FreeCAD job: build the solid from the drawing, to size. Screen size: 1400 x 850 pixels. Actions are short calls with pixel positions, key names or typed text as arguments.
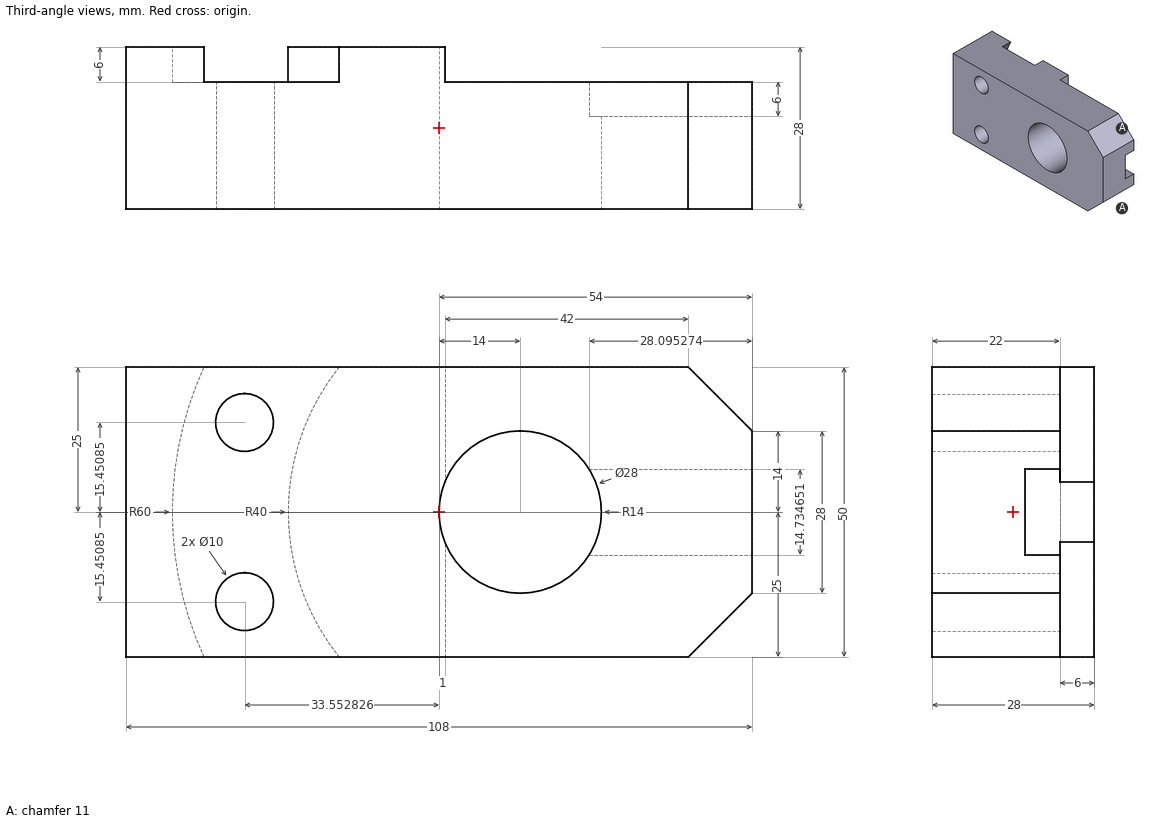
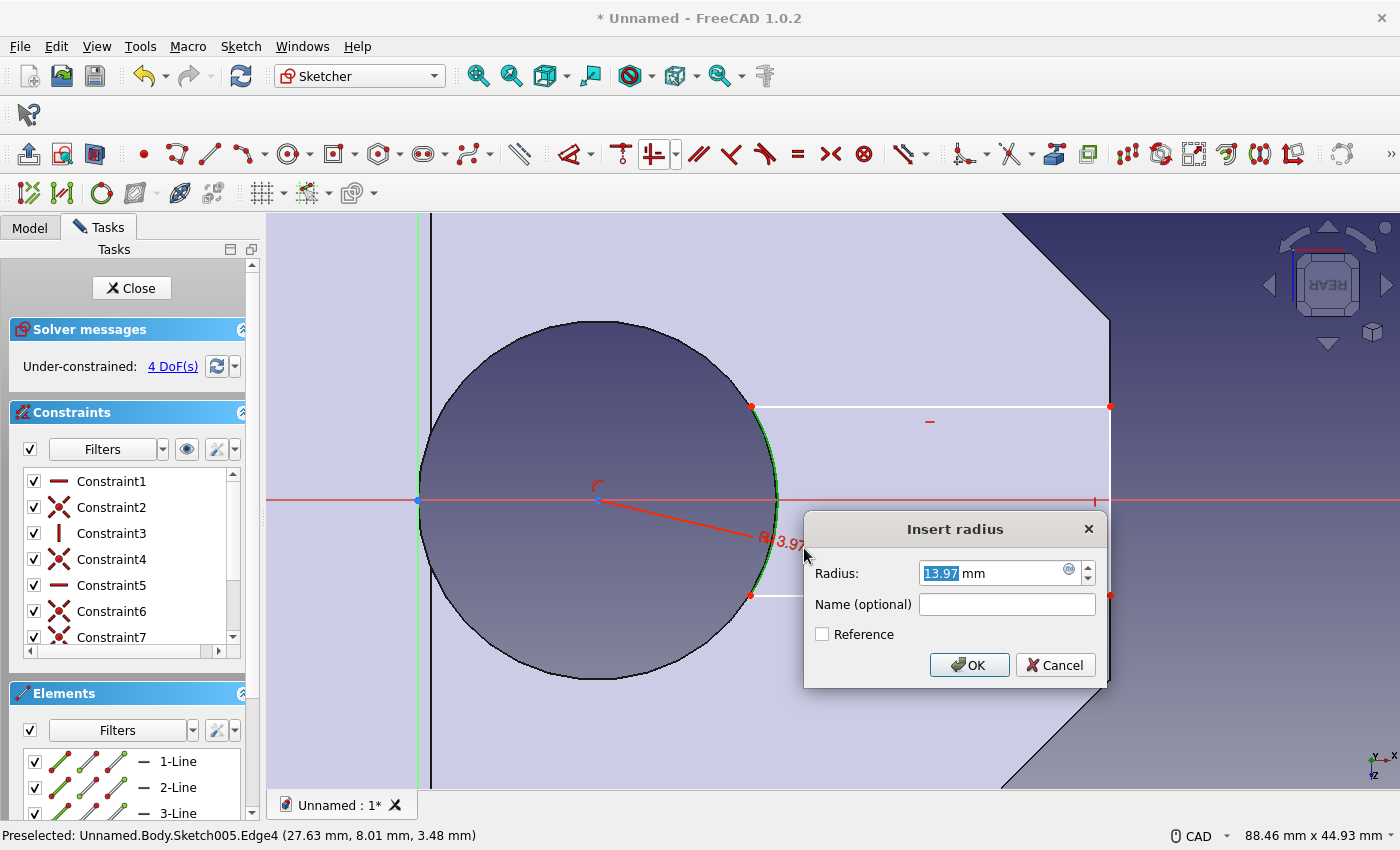
text(14)
key(Return)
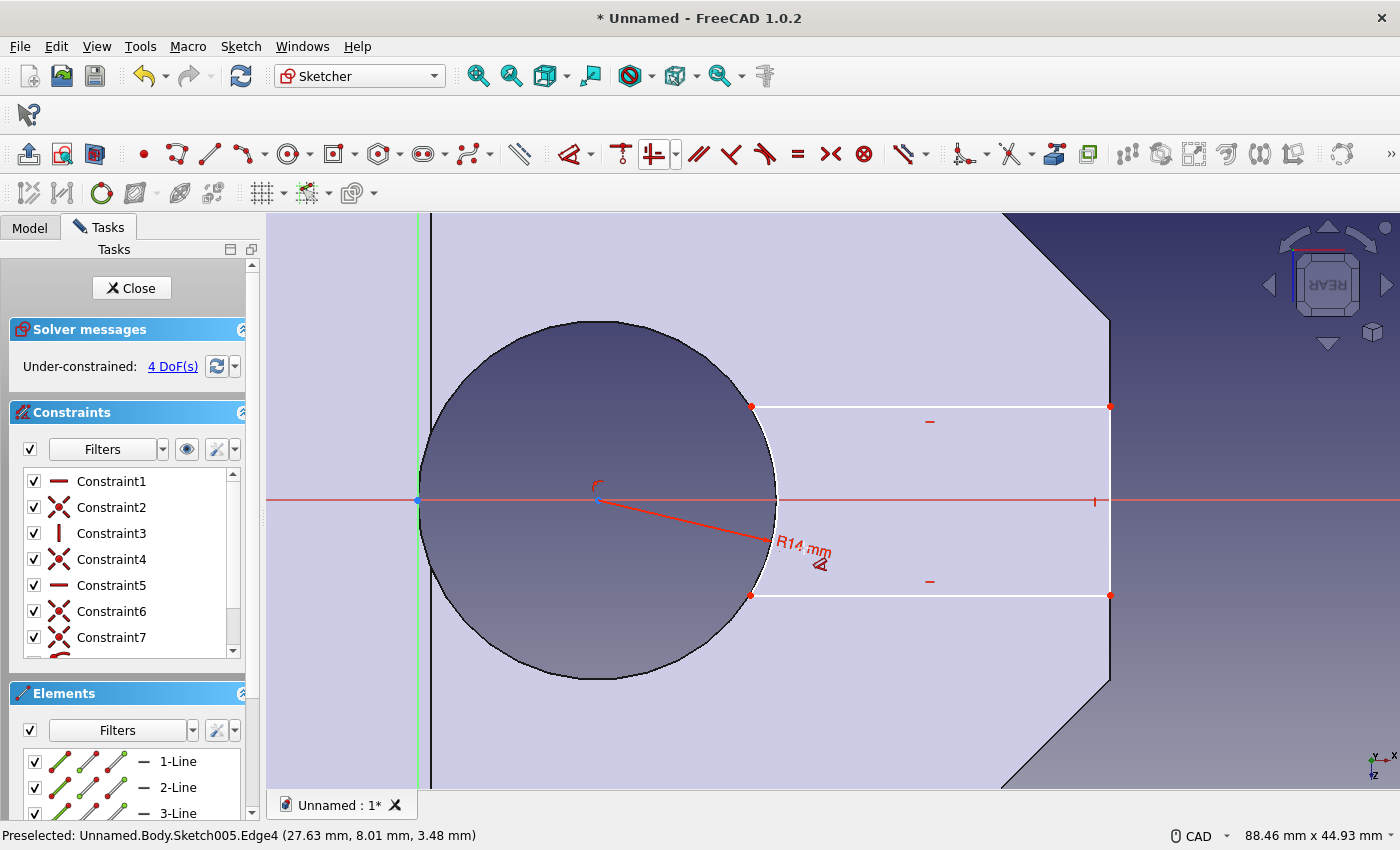
click(1110, 596)
click(764, 630)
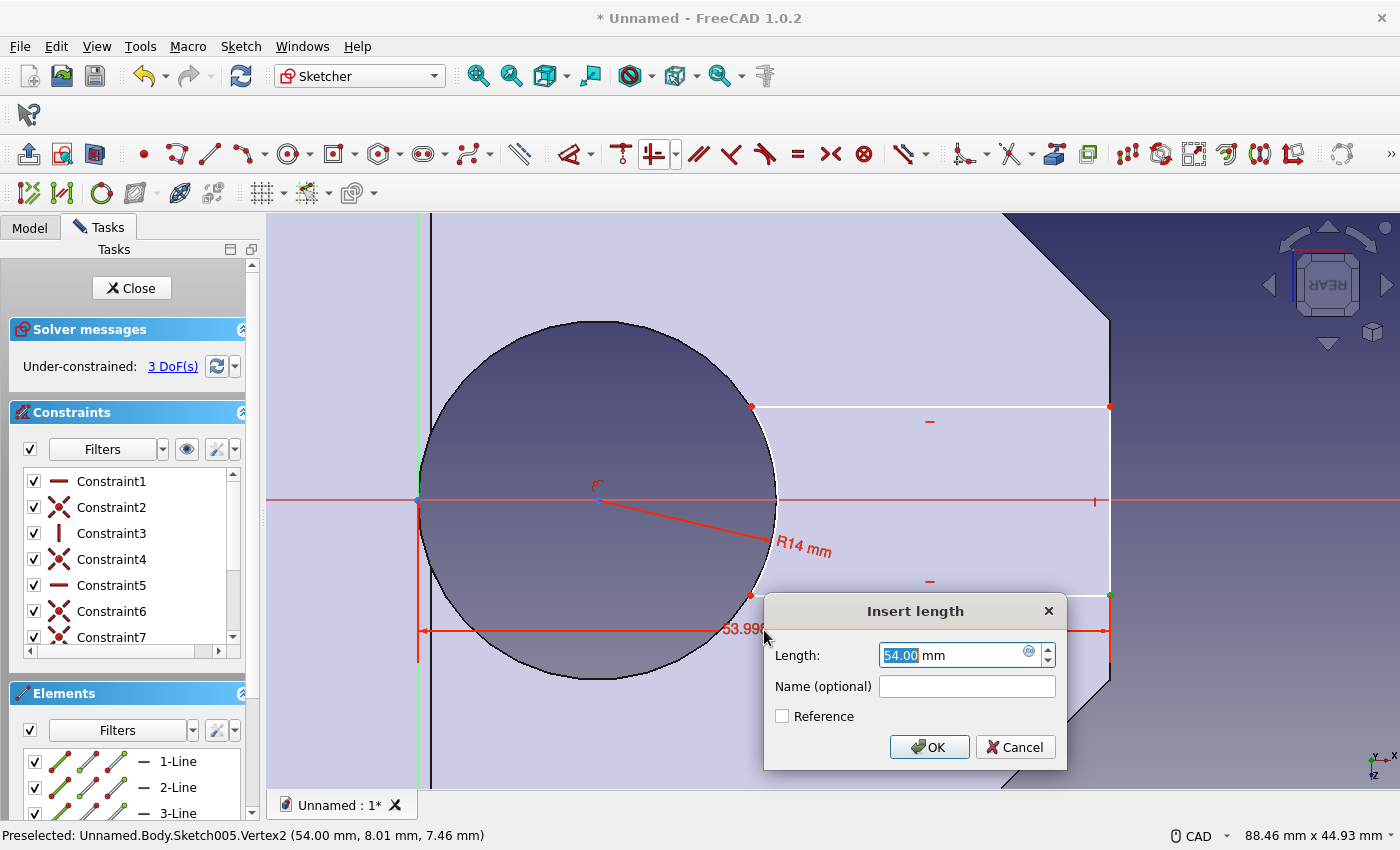
text(54)
key(Return)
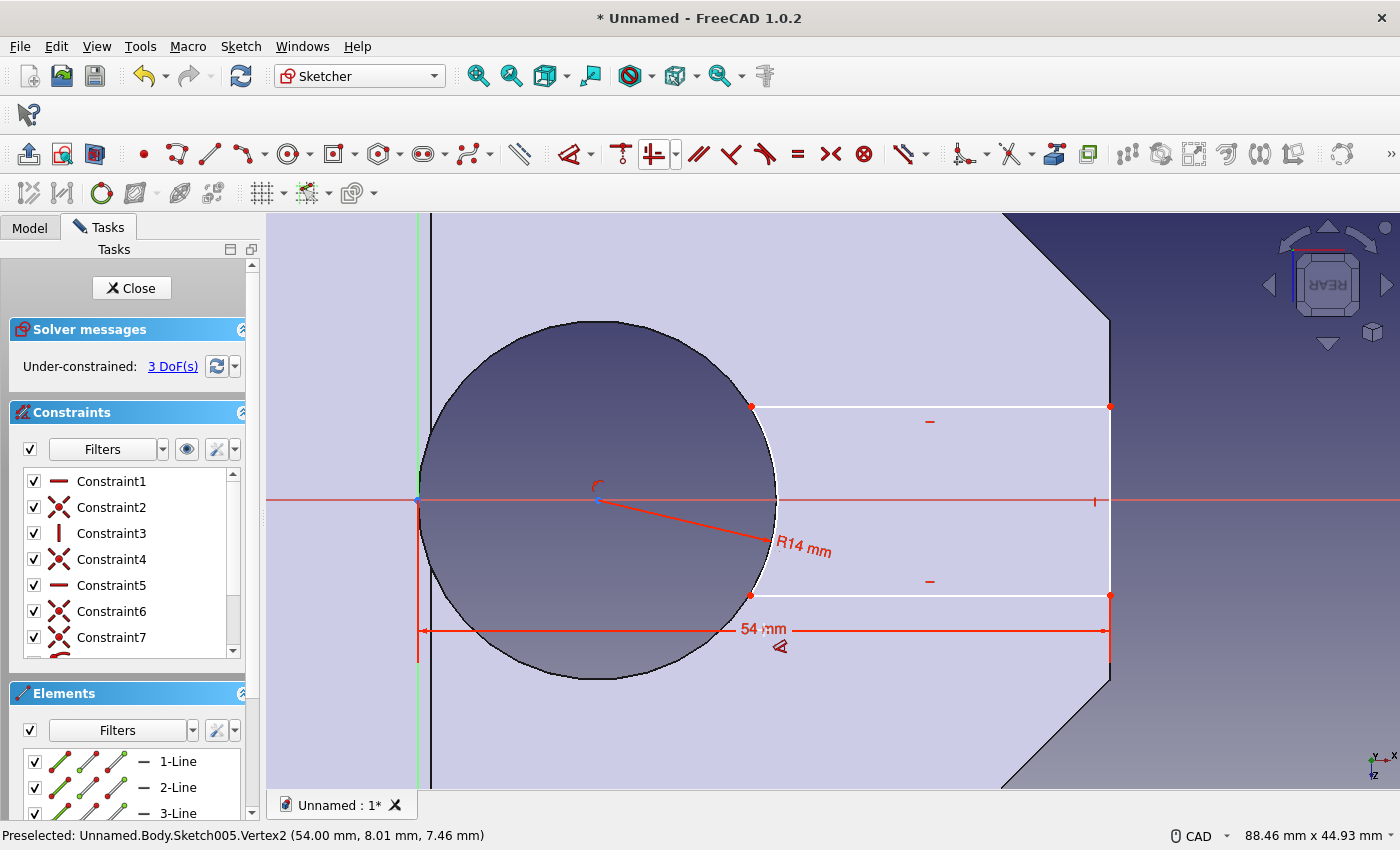
click(598, 500)
click(508, 534)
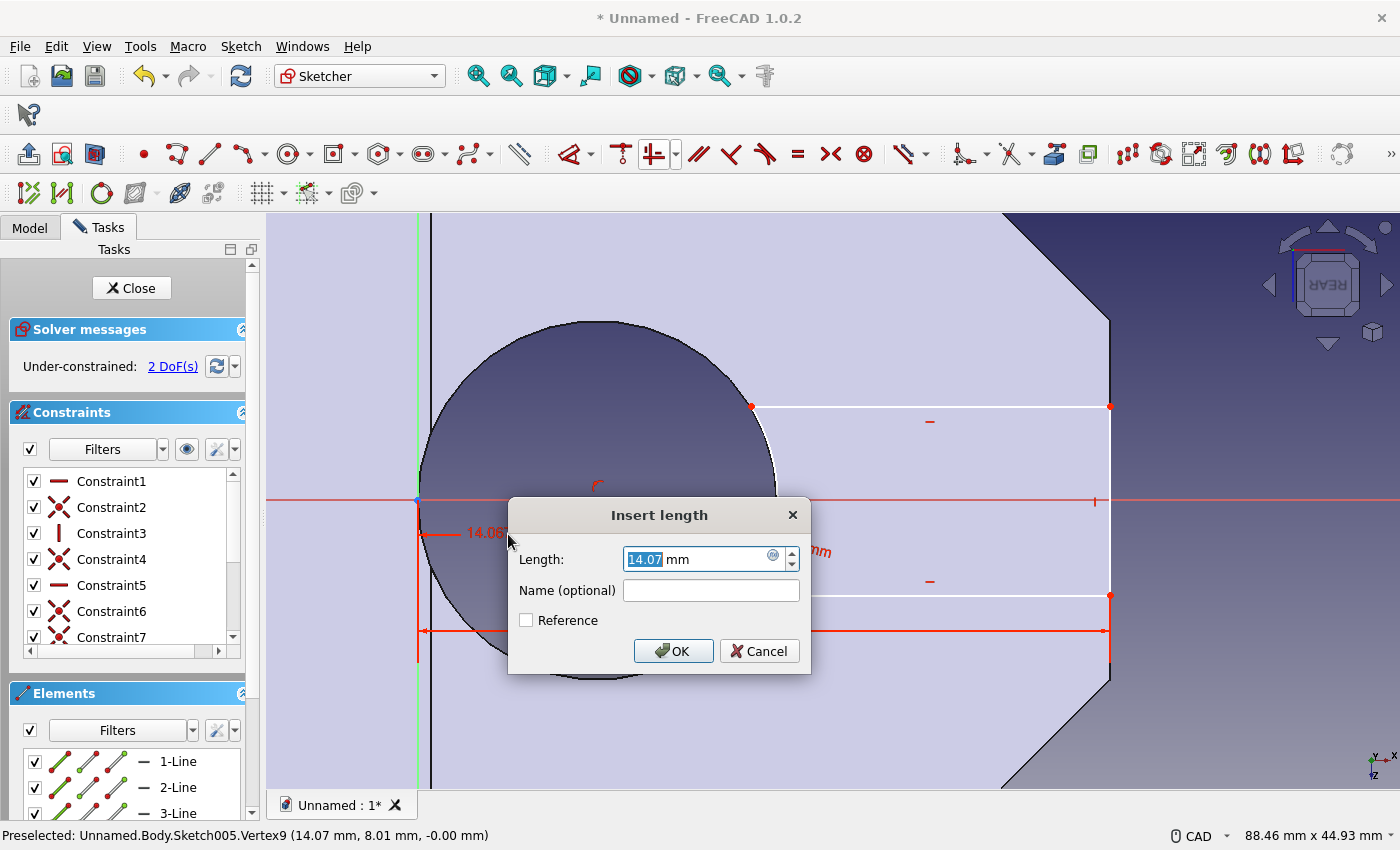
text(14)
key(Return)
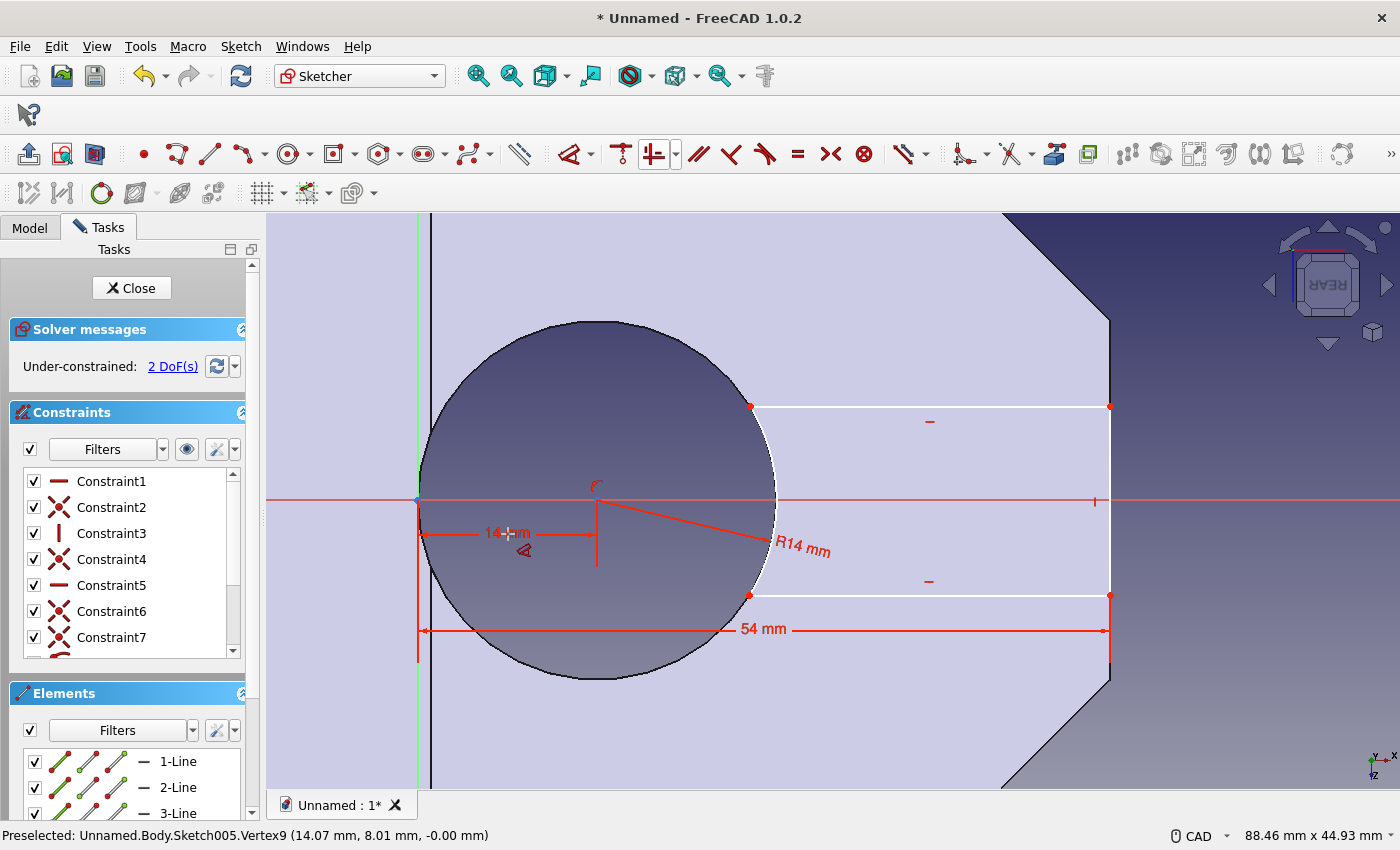
click(857, 596)
click(930, 630)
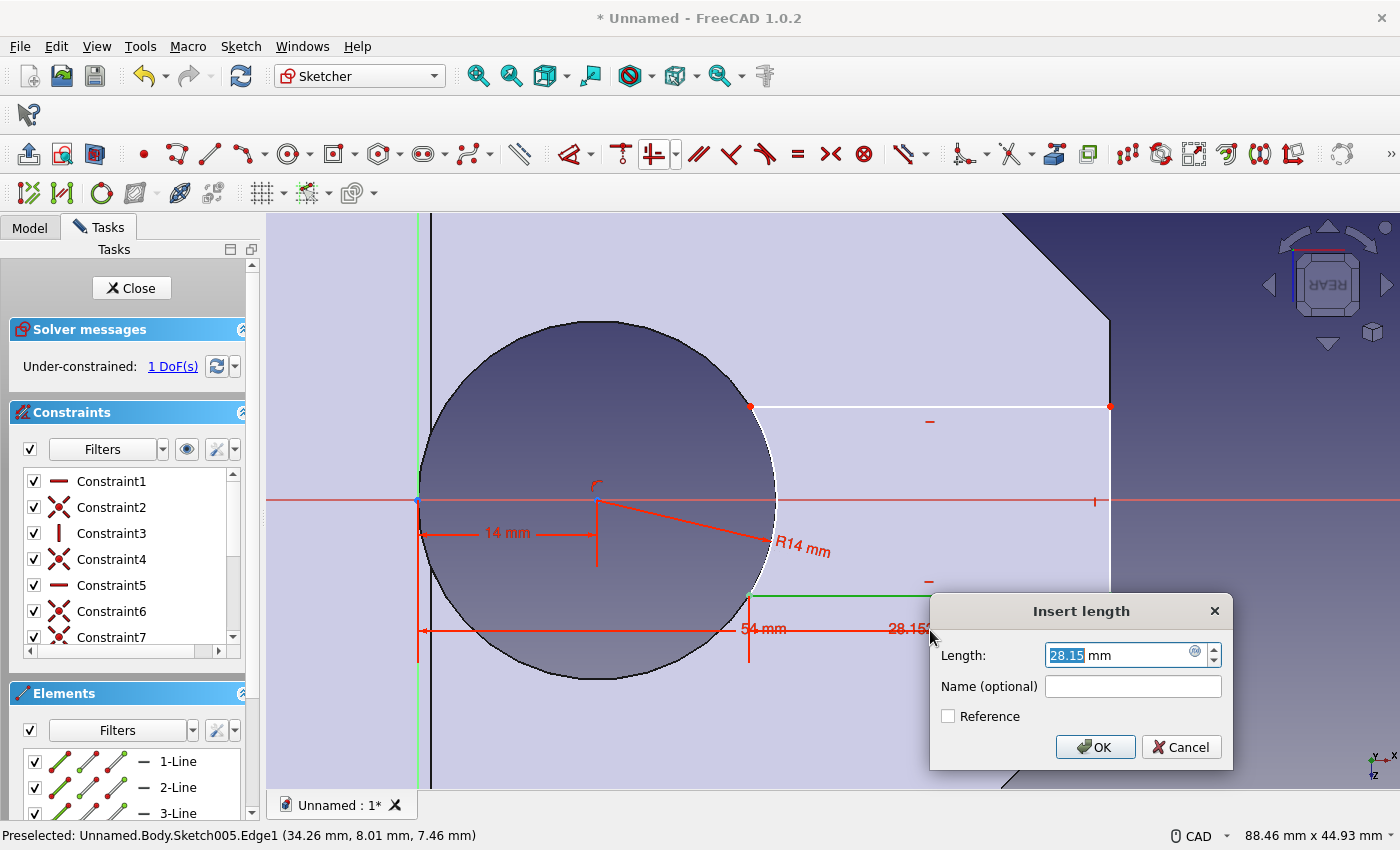
text(28.095274)
key(Return)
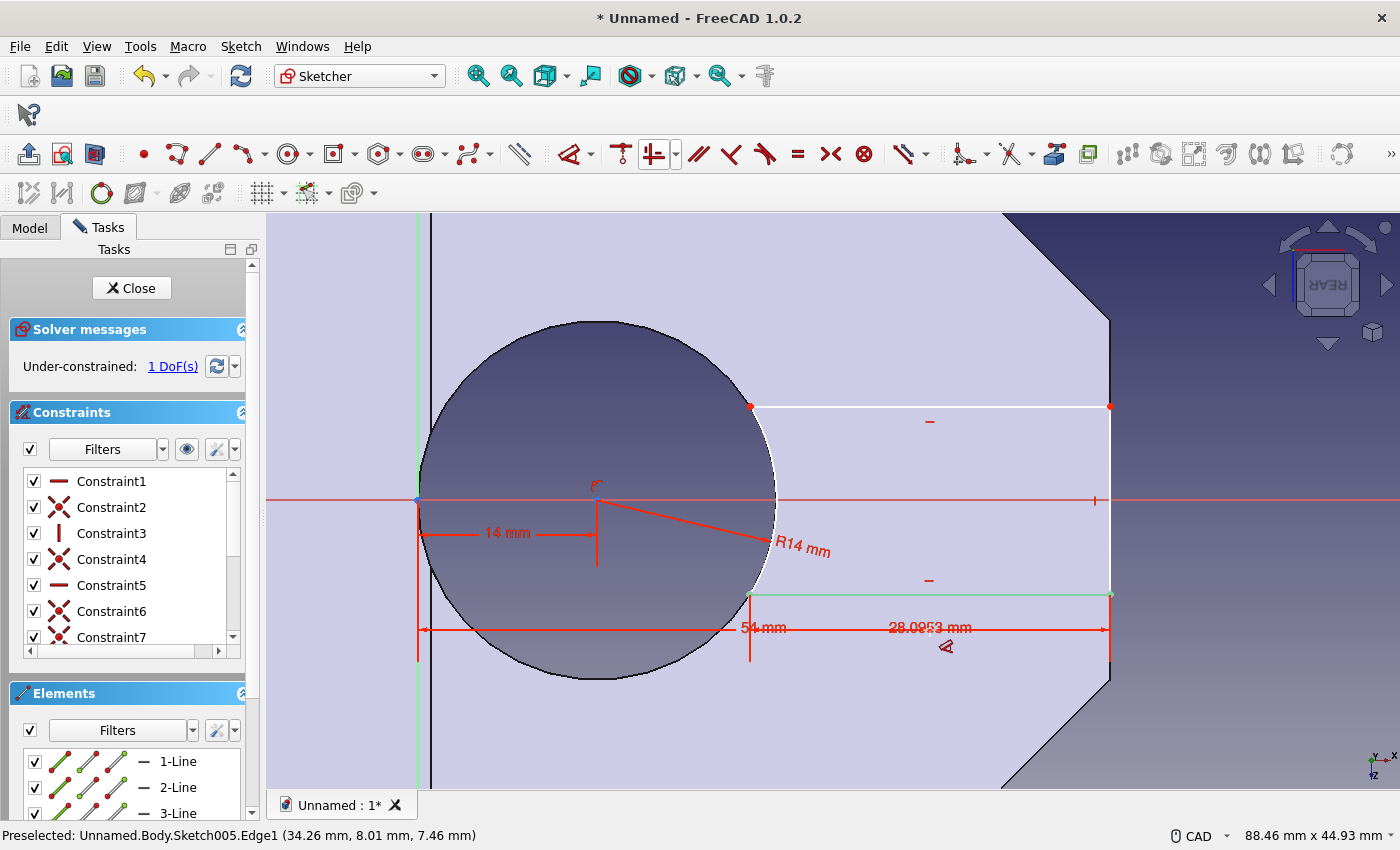
click(1110, 538)
click(1144, 458)